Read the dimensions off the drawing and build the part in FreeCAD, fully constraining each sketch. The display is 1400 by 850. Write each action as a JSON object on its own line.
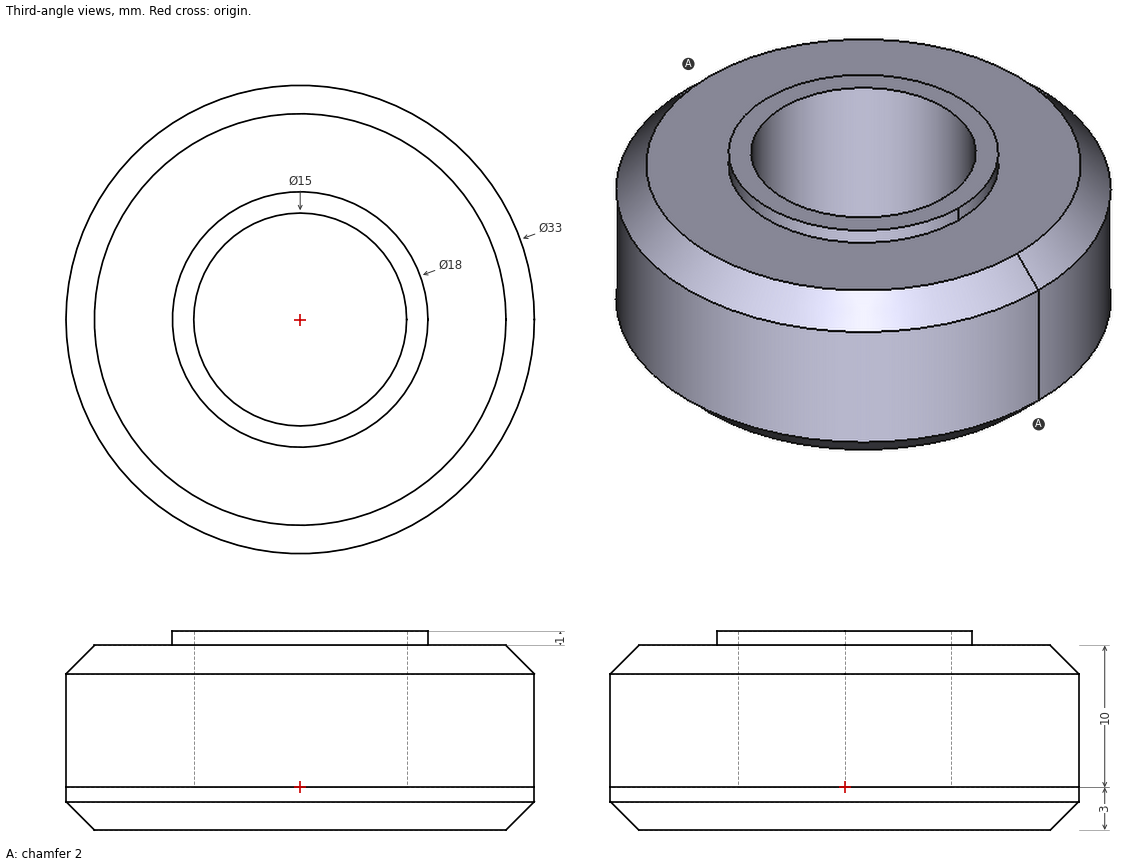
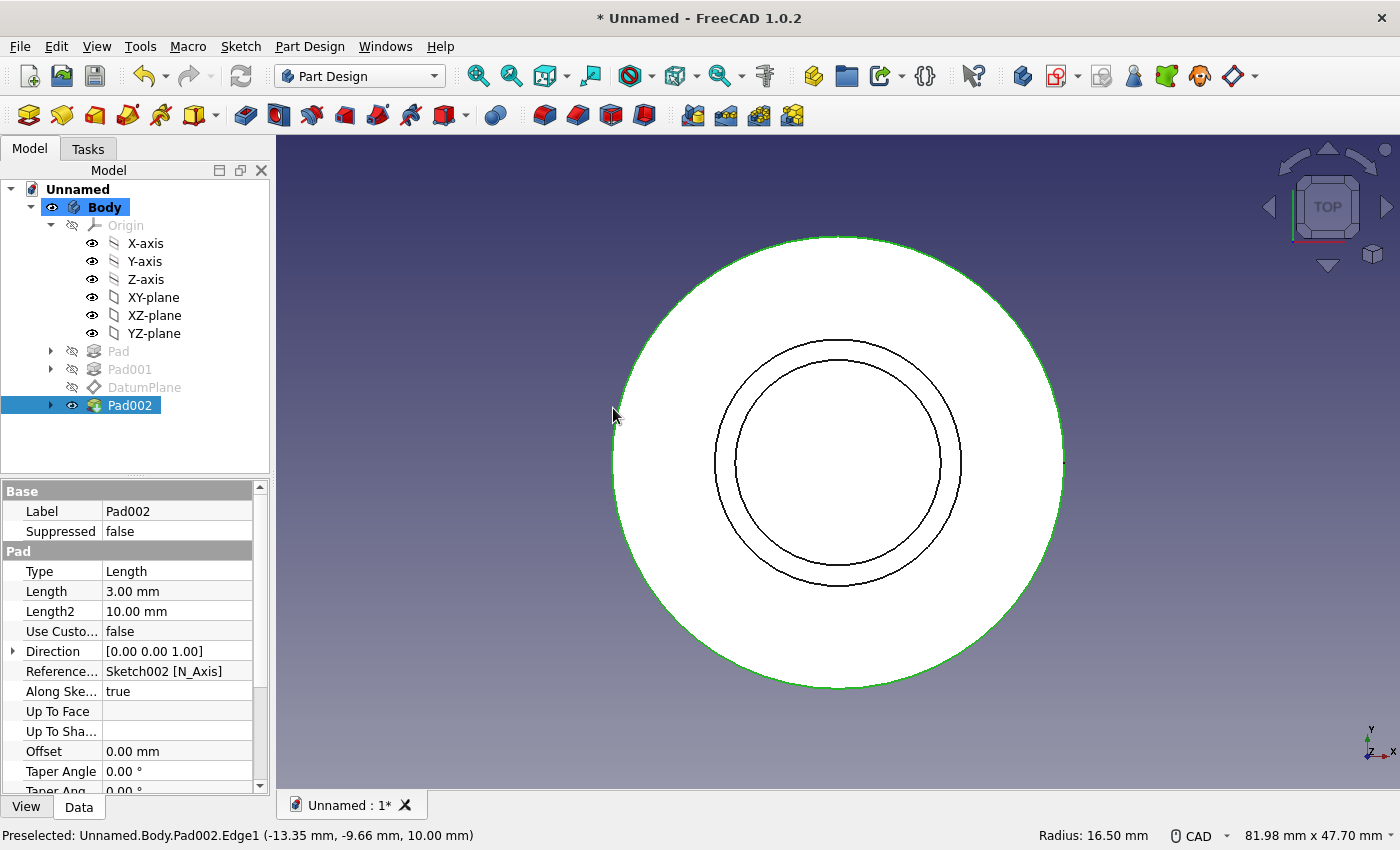
{"action": "key", "text": "1"}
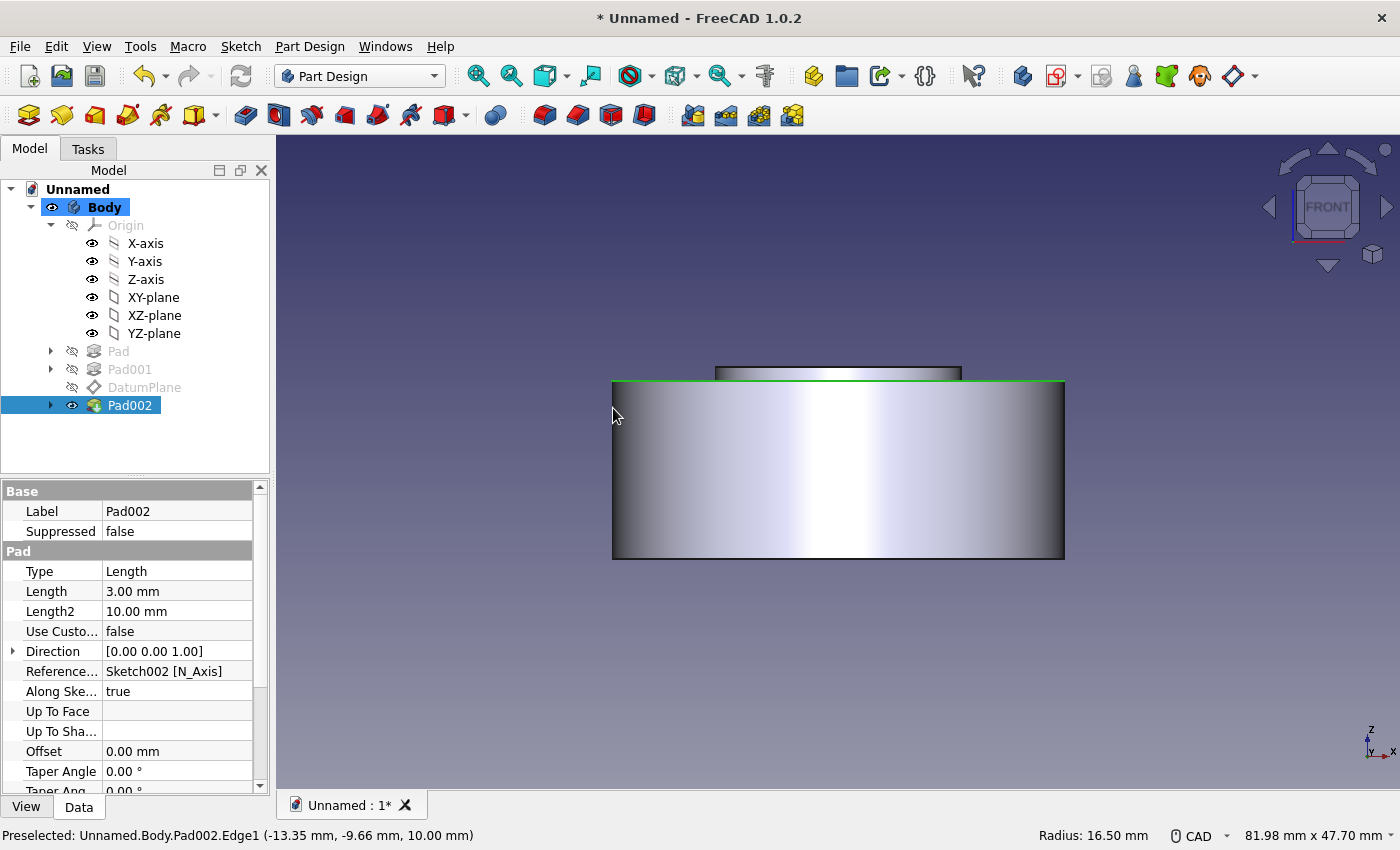
{"action": "key", "text": "v f"}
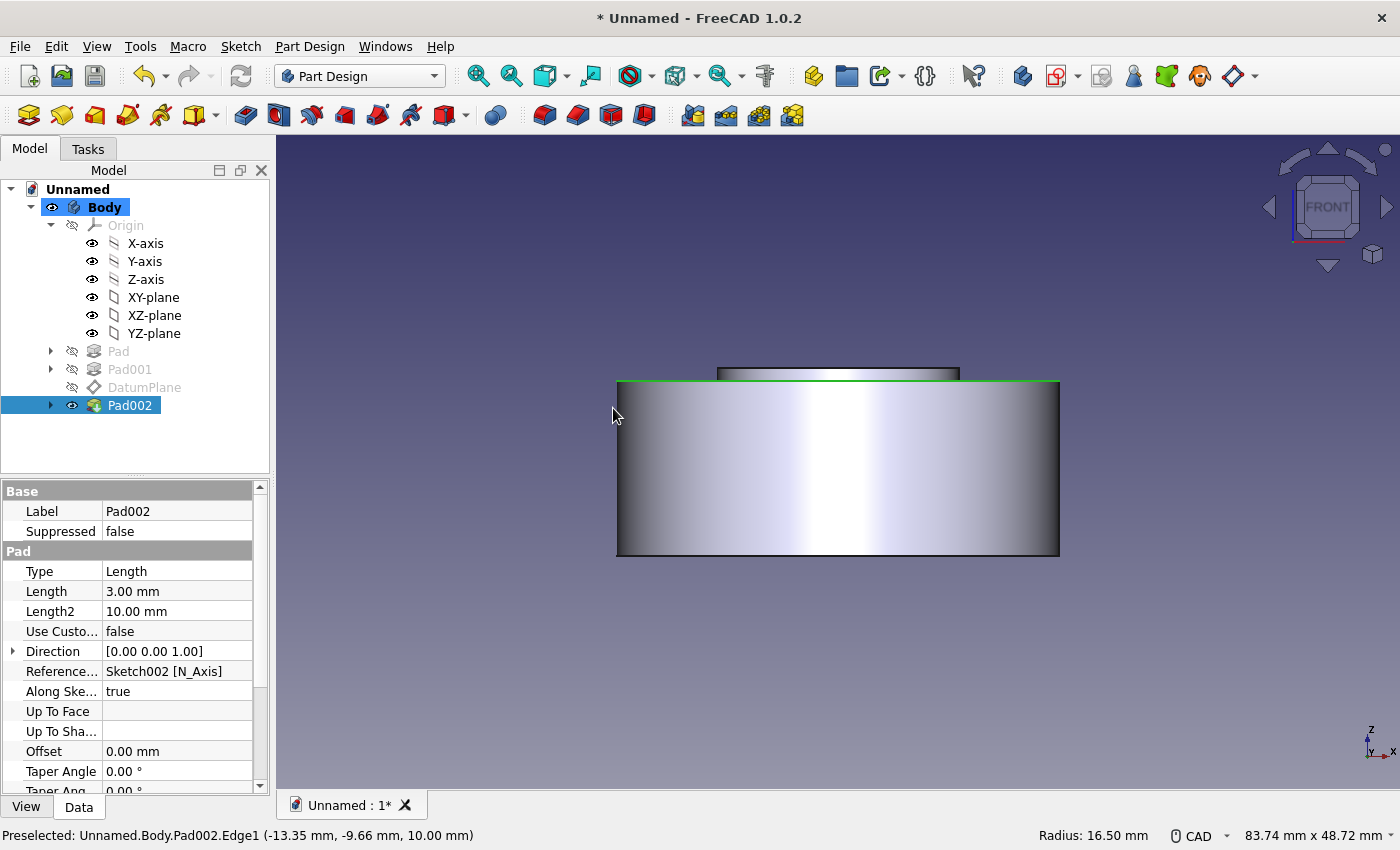
{"action": "left_click", "coordinate": [659, 555], "text": "ctrl"}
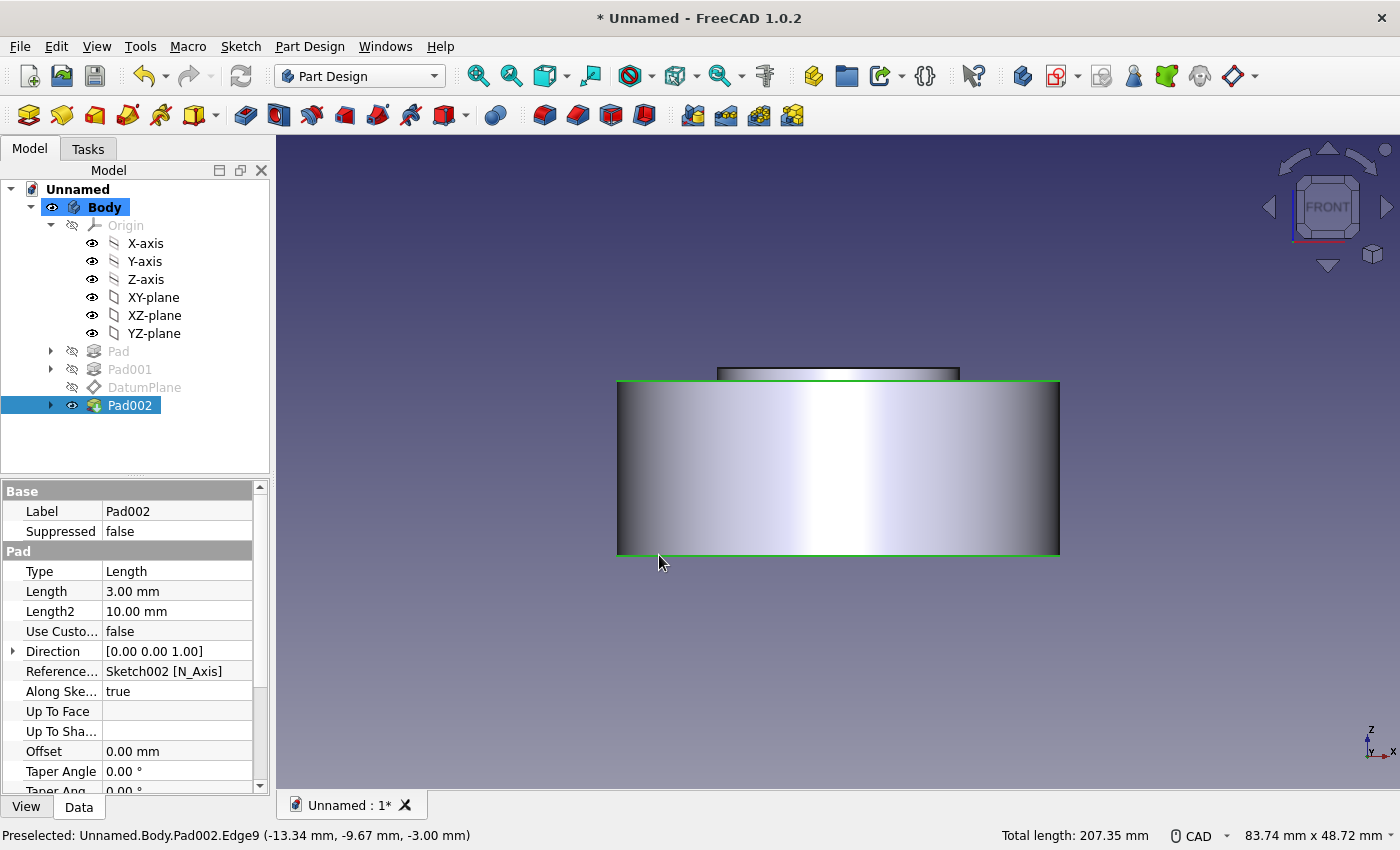
{"action": "left_click", "coordinate": [578, 116]}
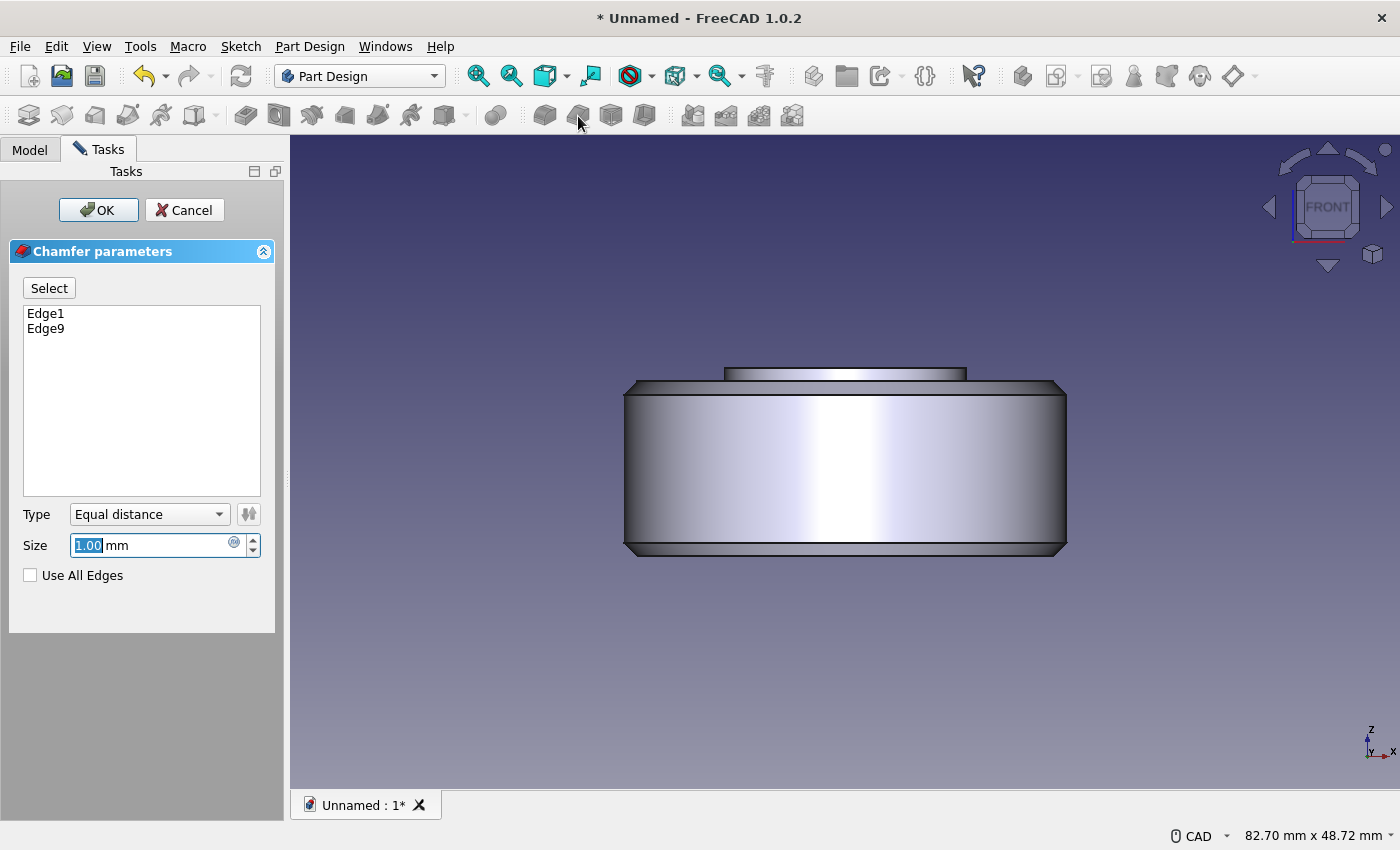
{"action": "type", "text": "2"}
{"action": "key", "text": "Tab"}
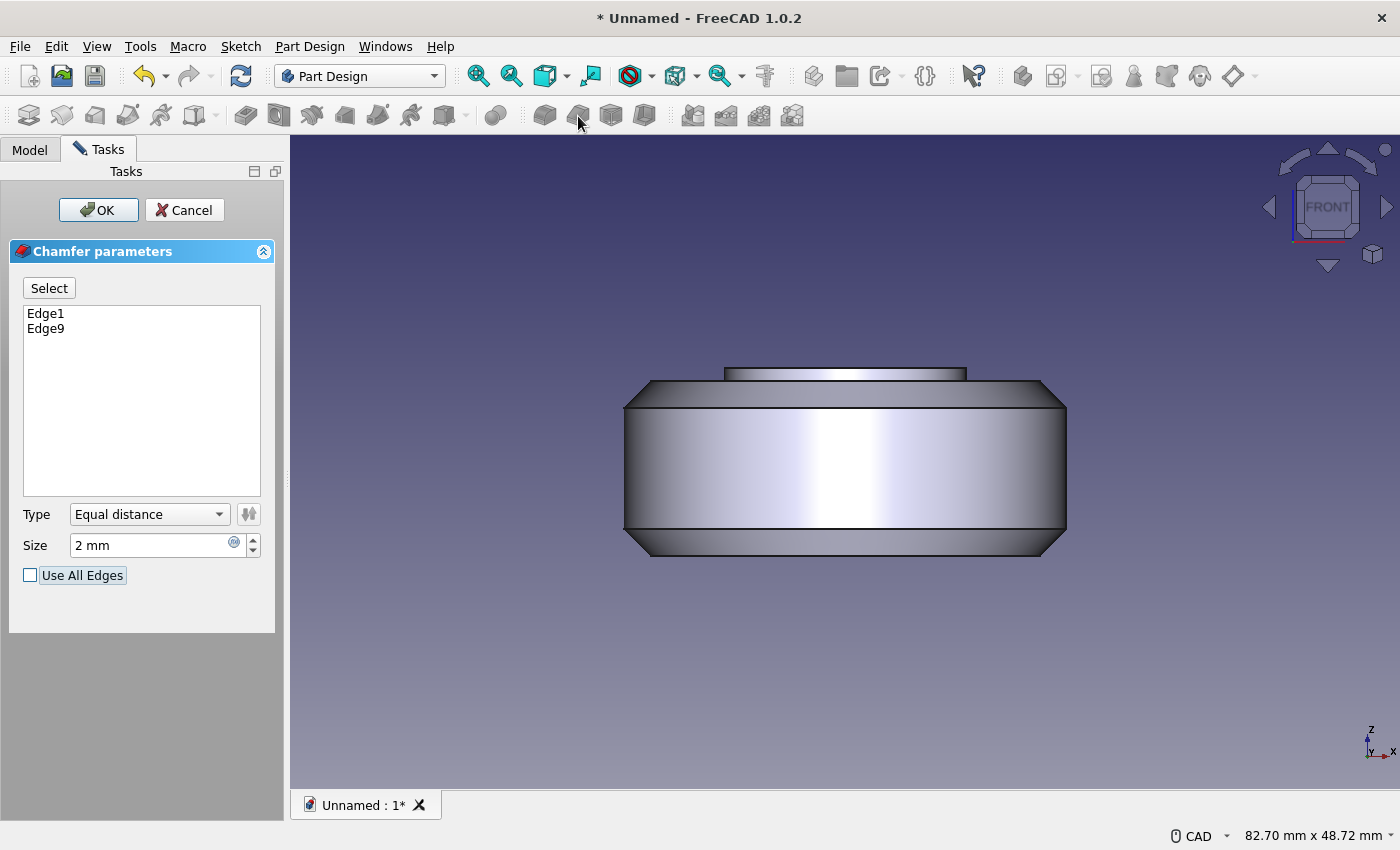
{"action": "left_click", "coordinate": [99, 210]}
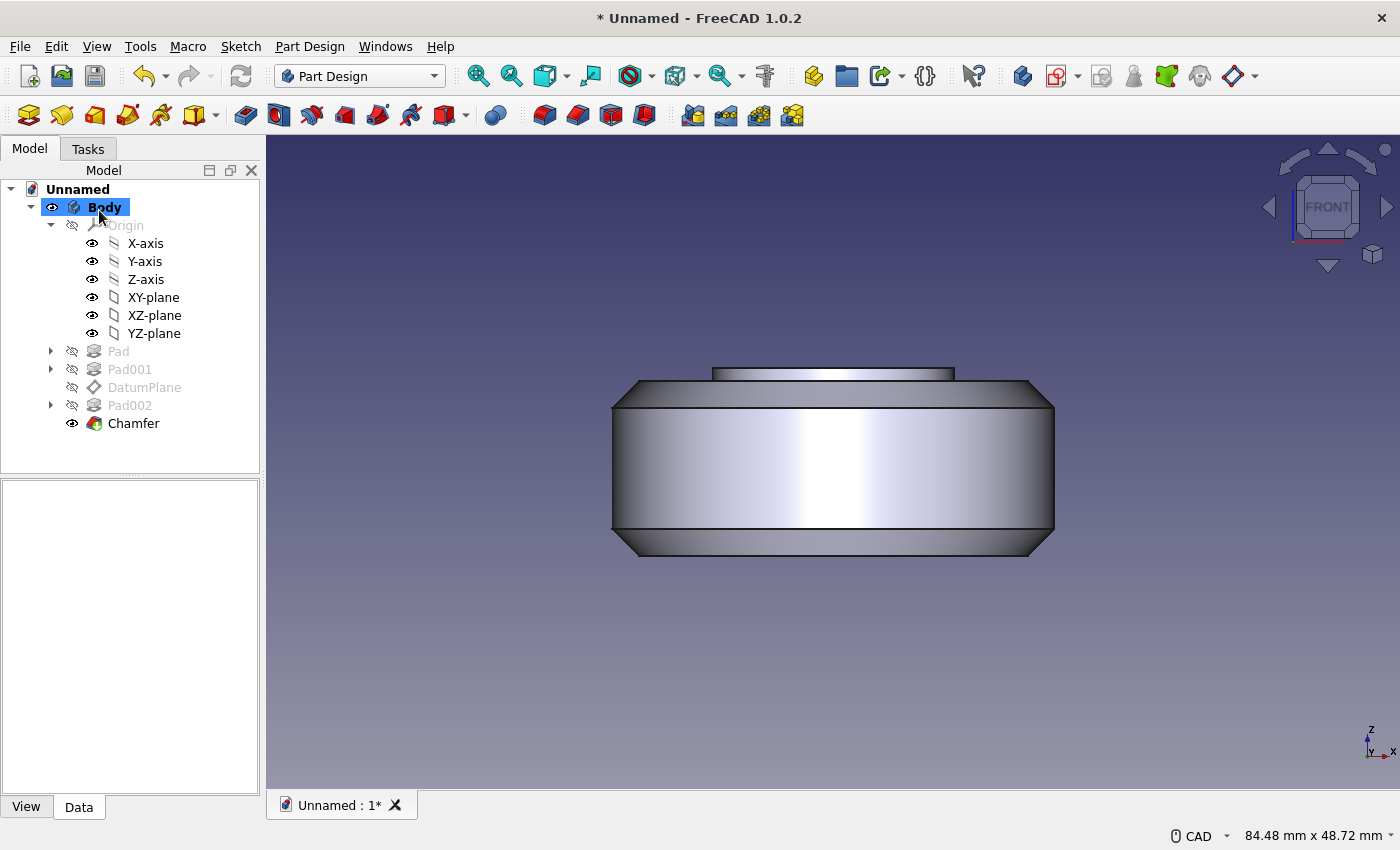
{"action": "key", "text": "0"}